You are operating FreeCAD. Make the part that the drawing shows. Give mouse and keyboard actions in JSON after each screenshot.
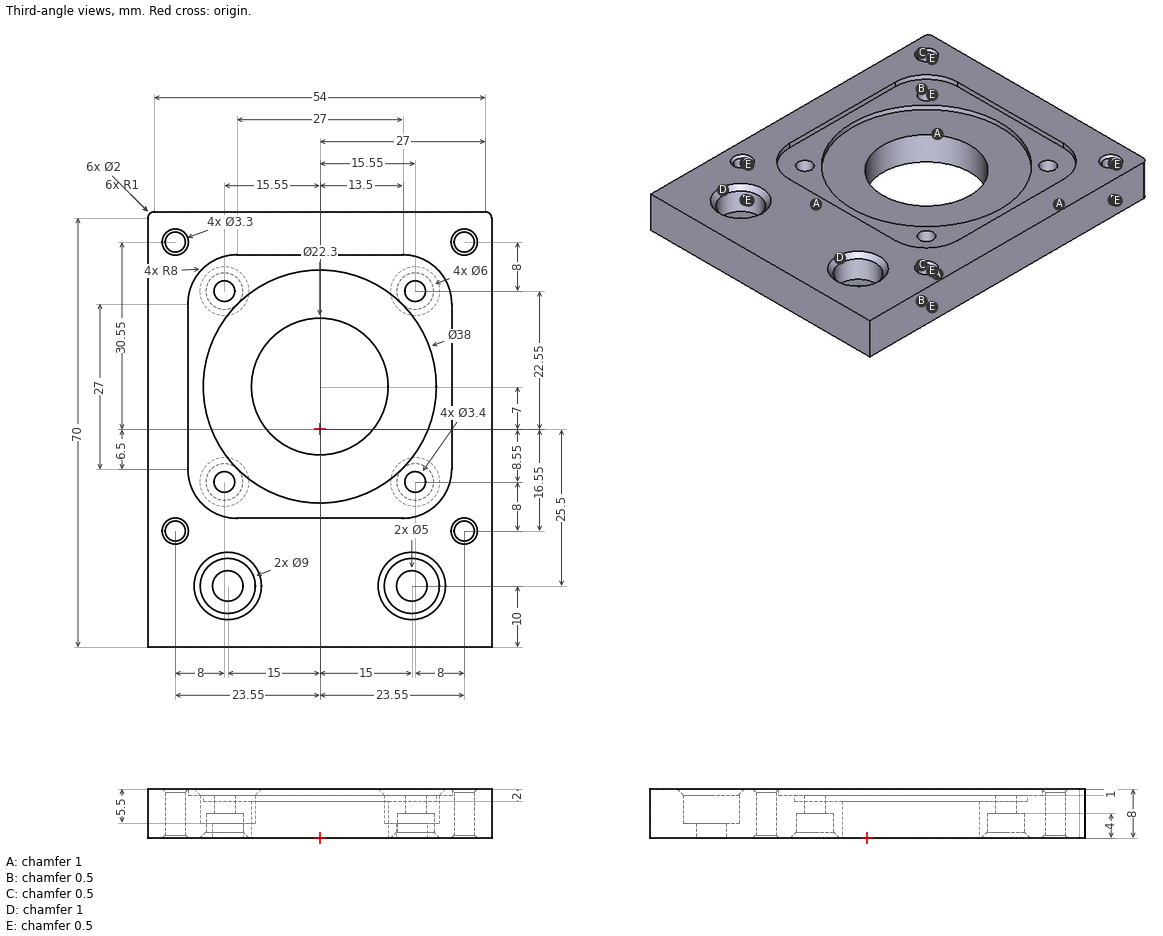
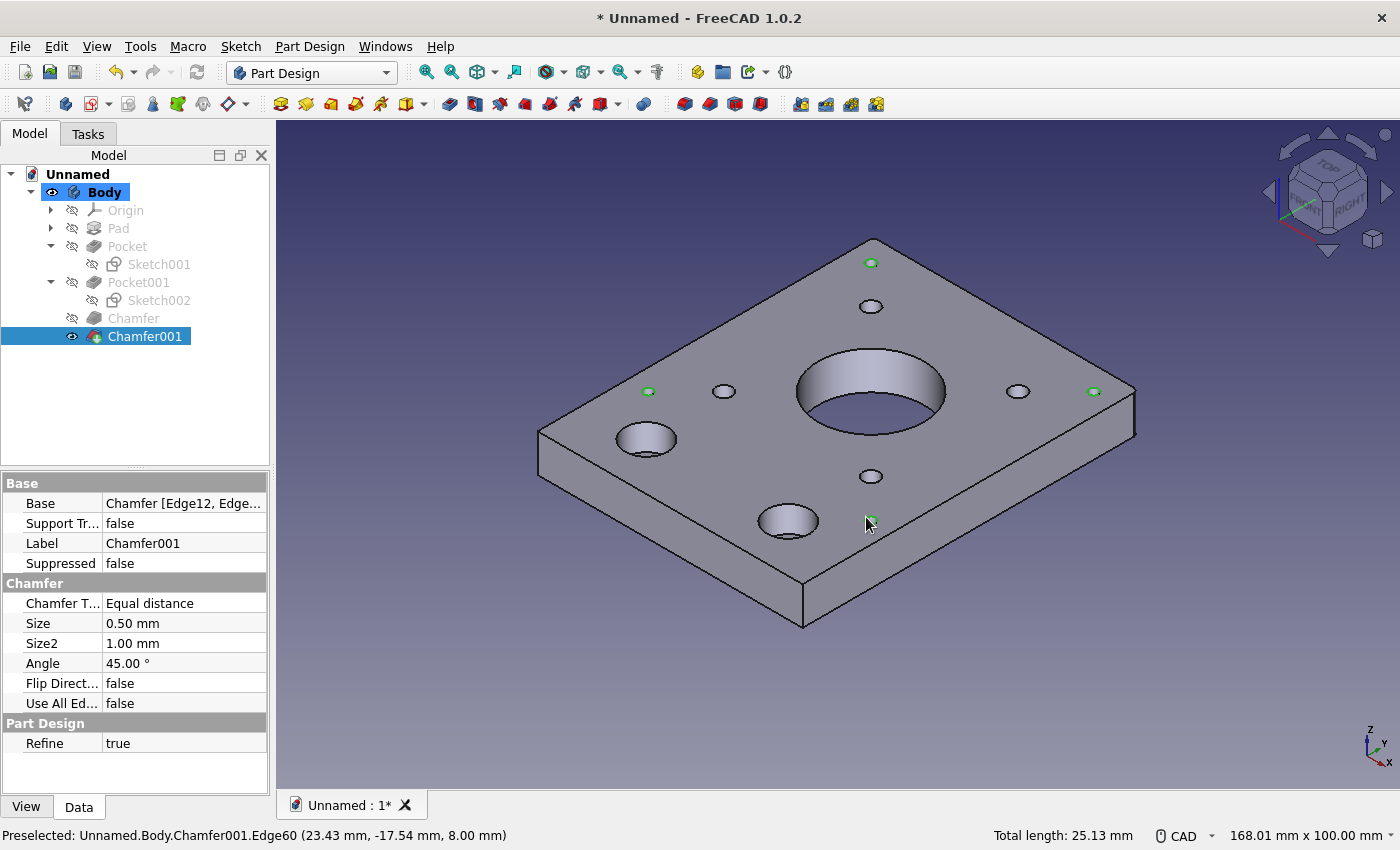
{"action": "left_click", "coordinate": [710, 104]}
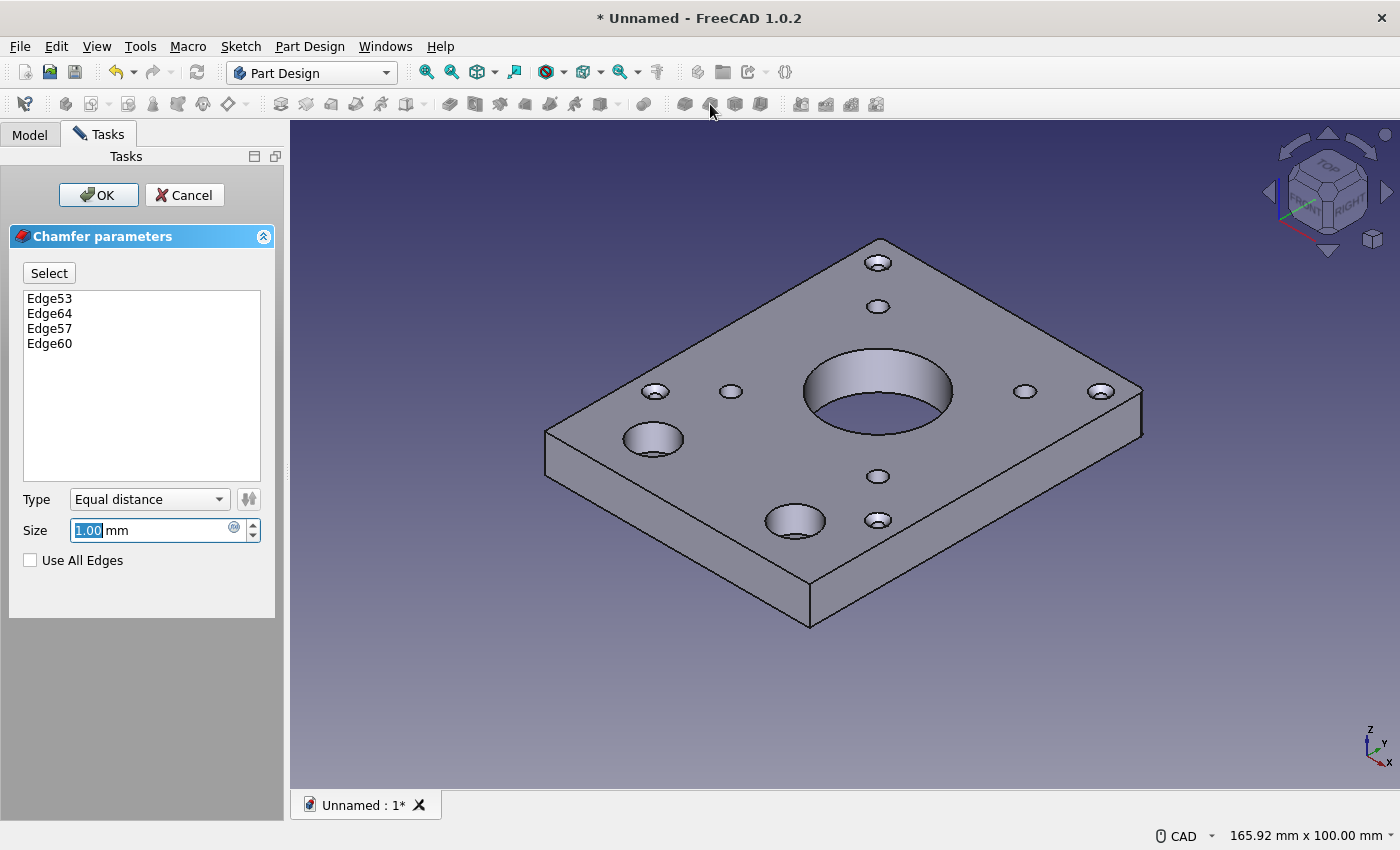
{"action": "type", "text": "0.5"}
{"action": "key", "text": "Tab"}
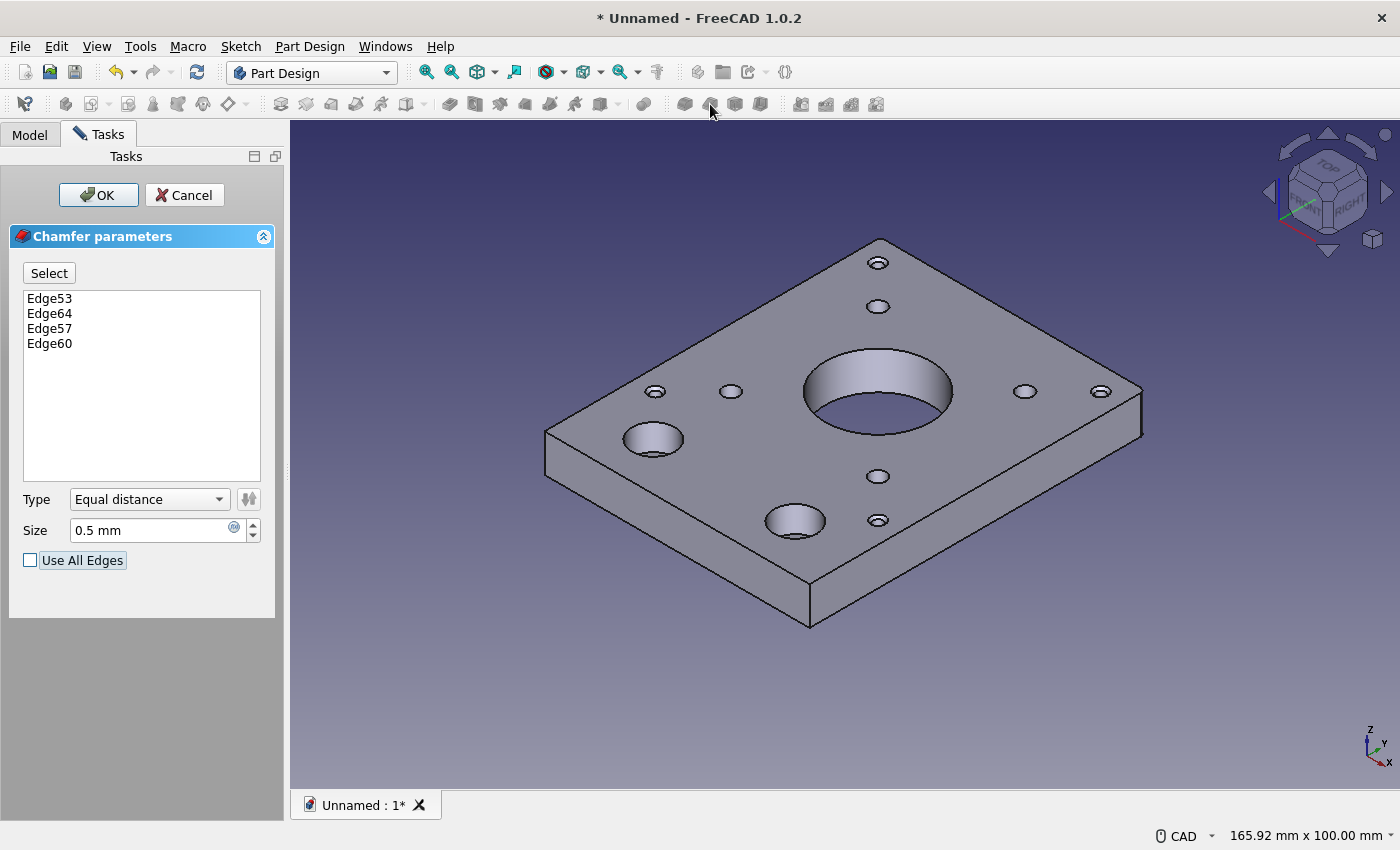
{"action": "left_click", "coordinate": [99, 195]}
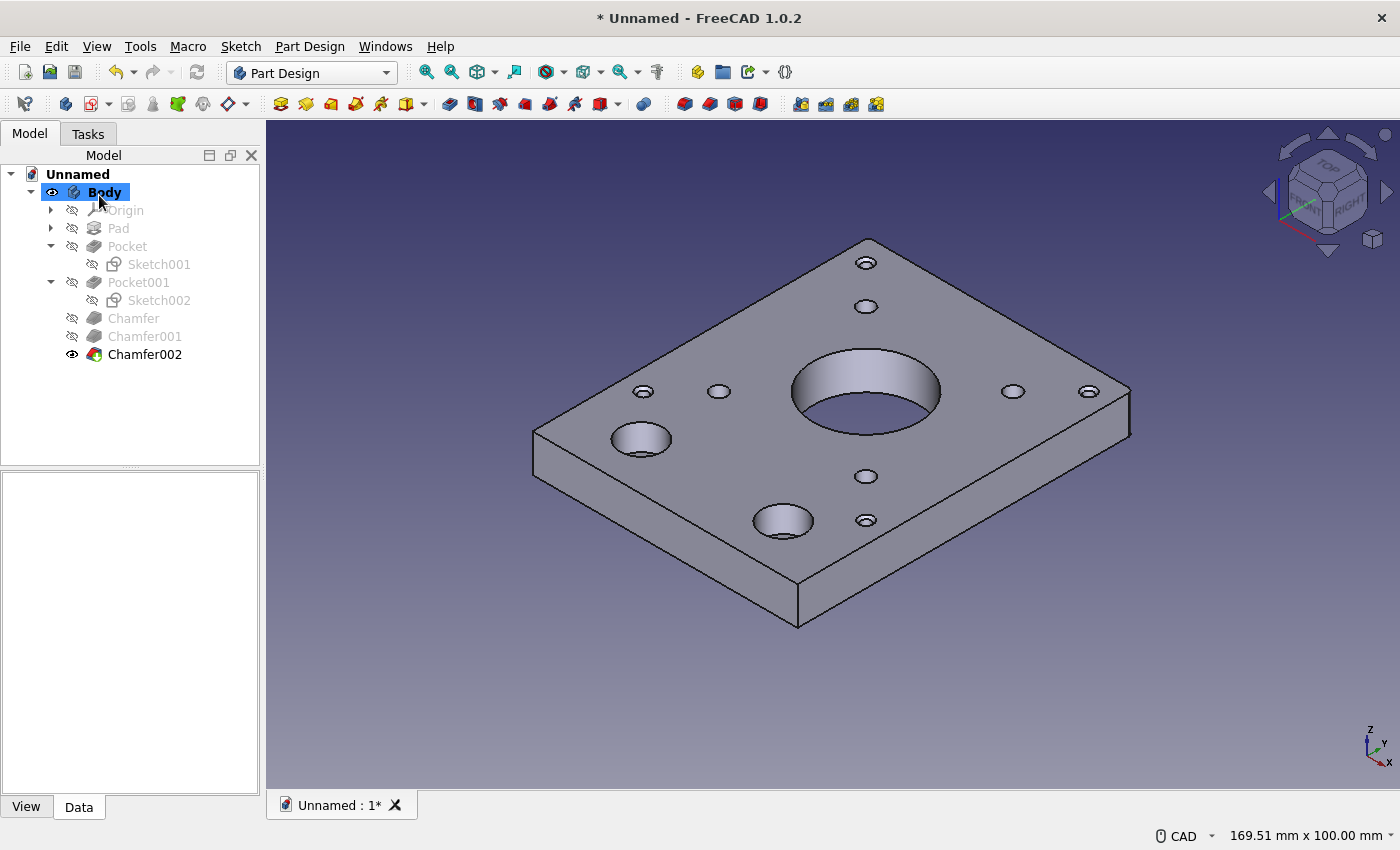
{"action": "left_click", "coordinate": [737, 465]}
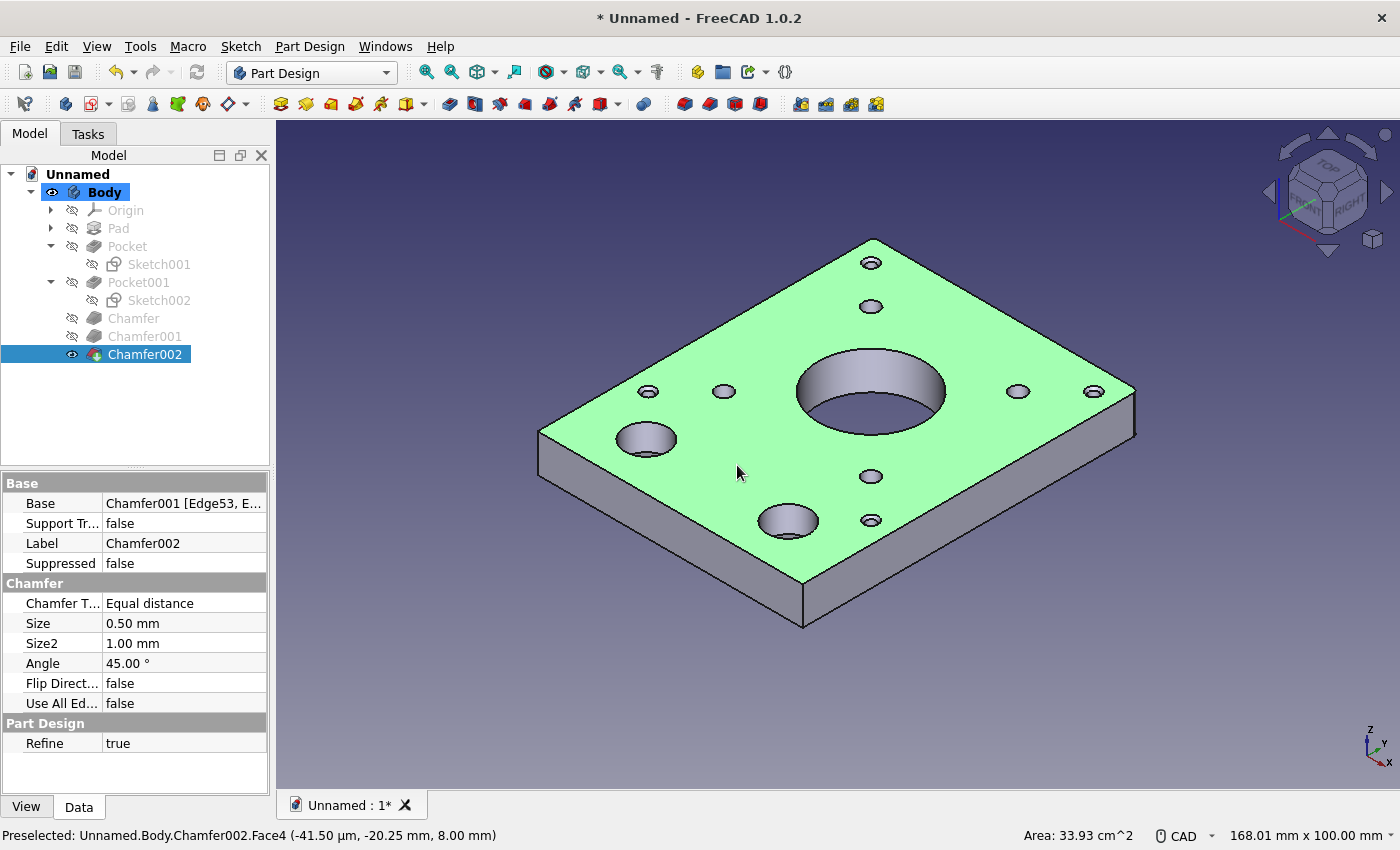
{"action": "left_click", "coordinate": [90, 104]}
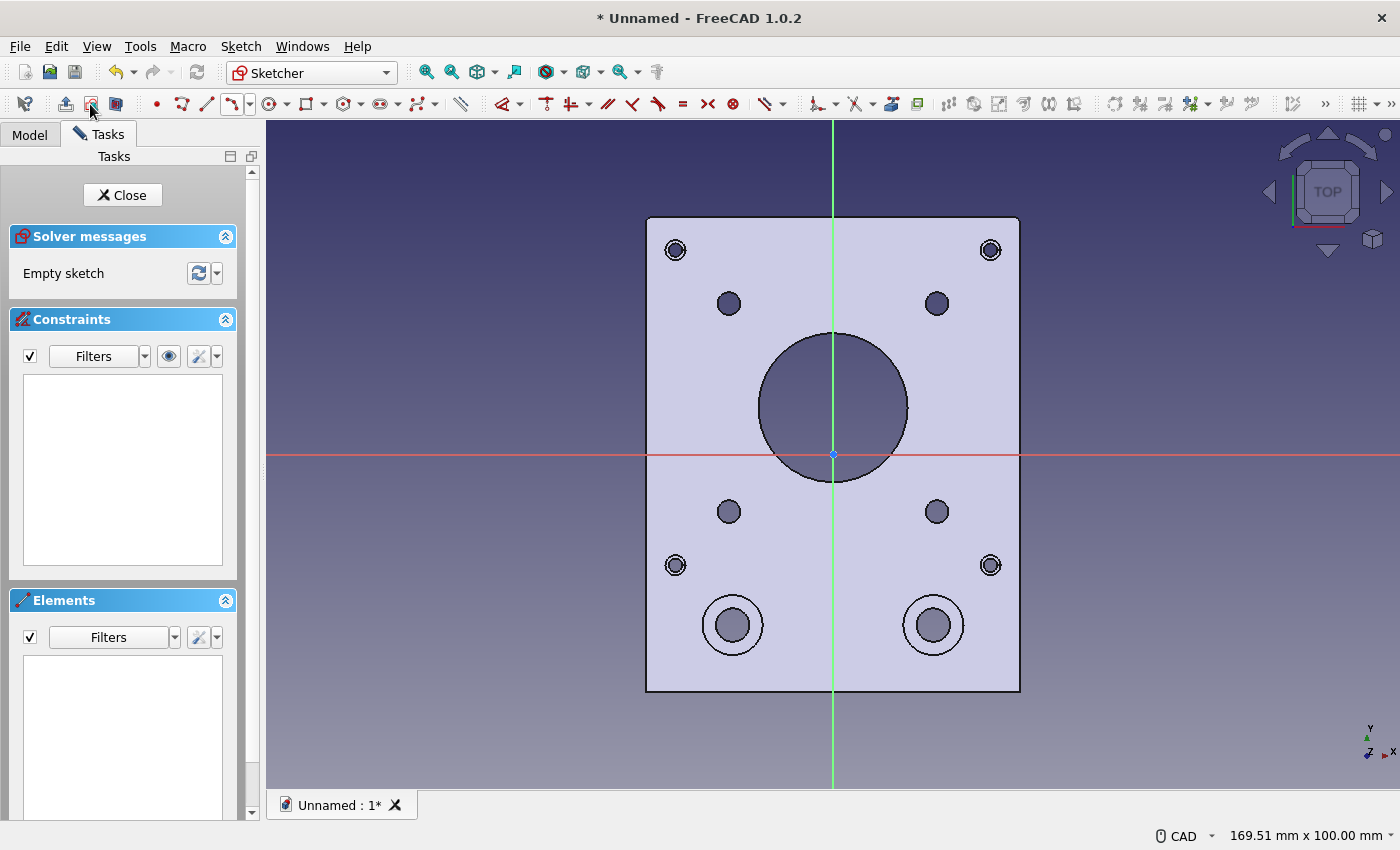
{"action": "scroll", "coordinate": [916, 351], "scroll_direction": "up", "scroll_amount": 3}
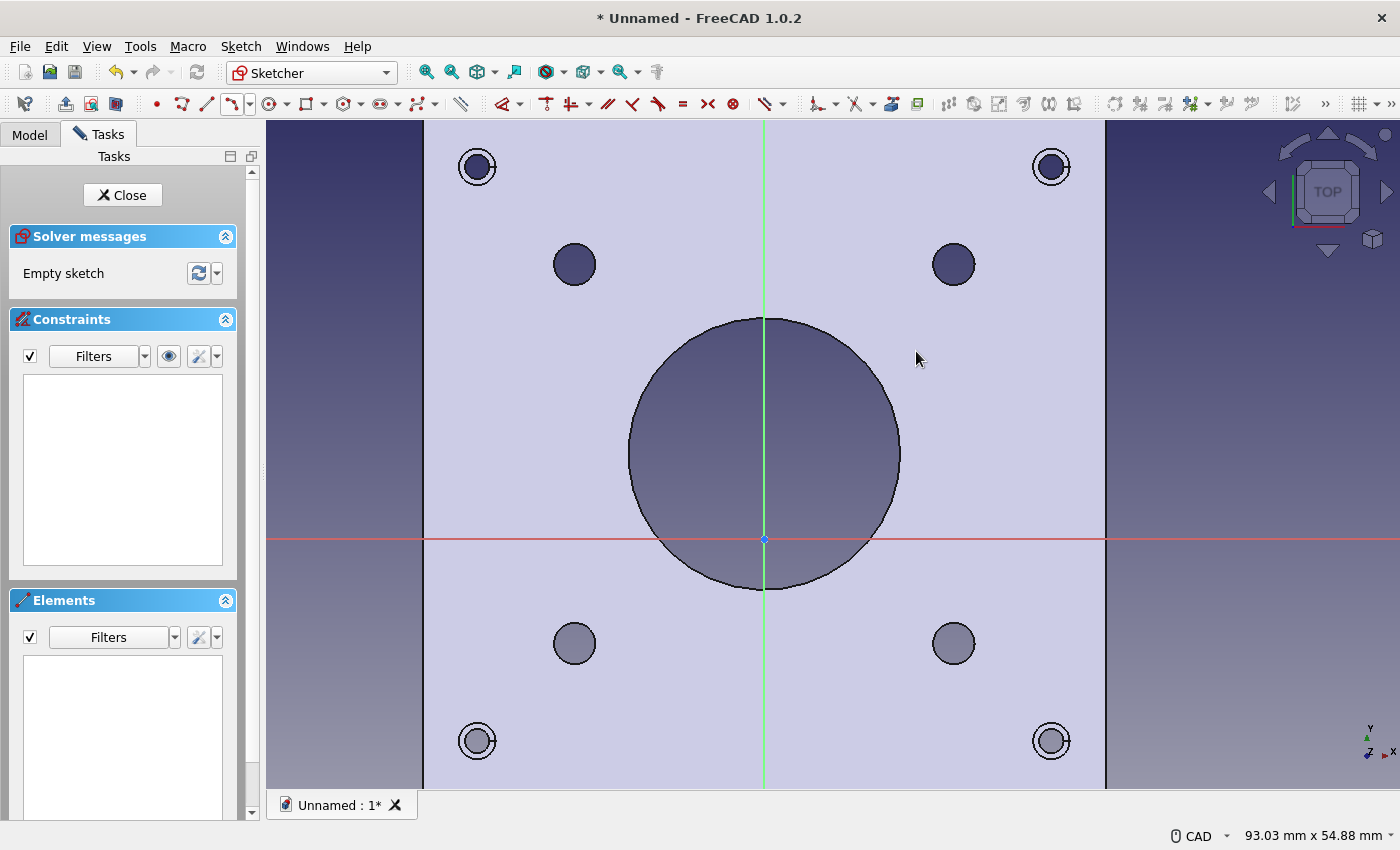
{"action": "left_click", "coordinate": [268, 104]}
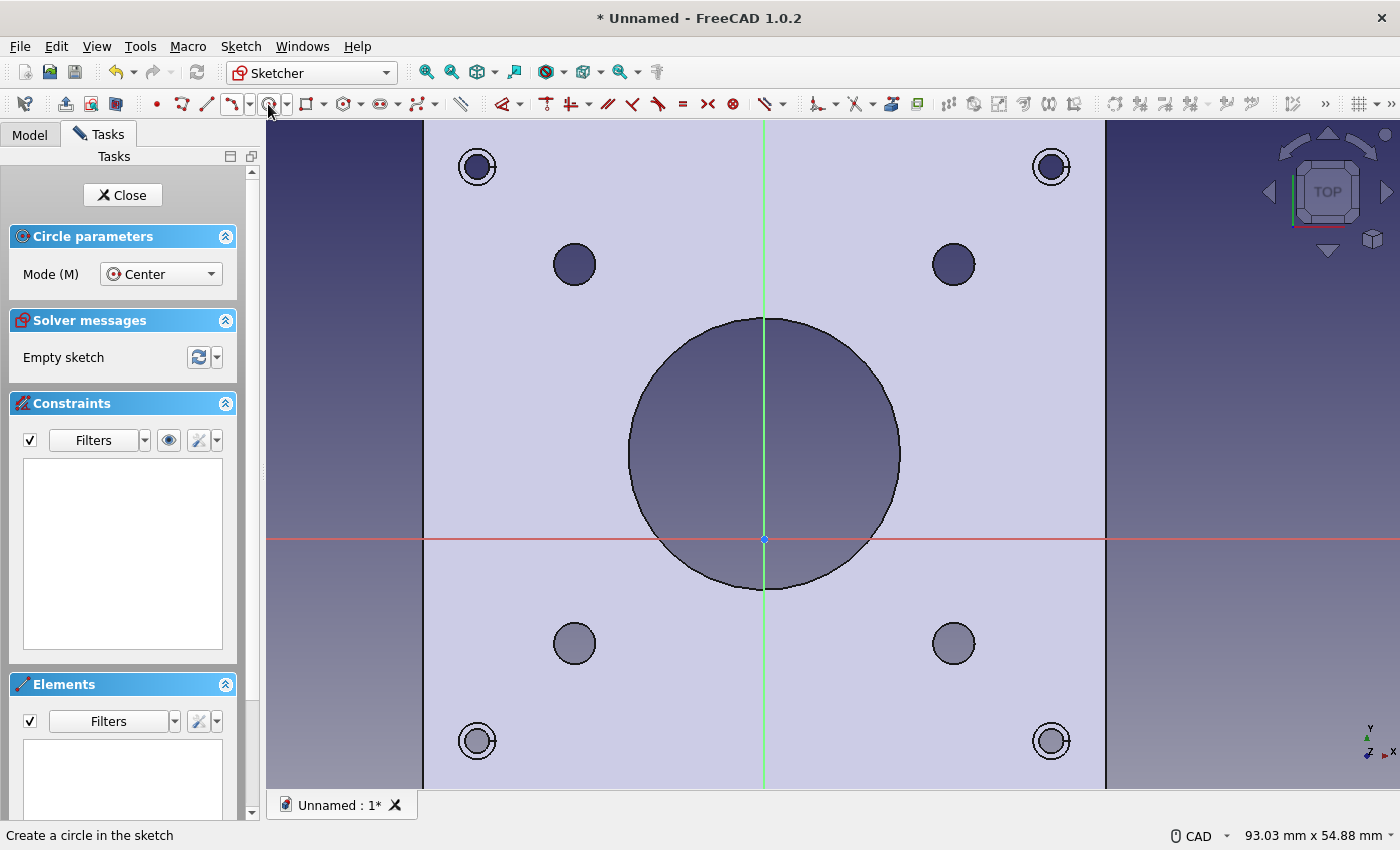
{"action": "left_click", "coordinate": [764, 454]}
{"action": "left_click", "coordinate": [928, 290]}
{"action": "key", "text": "Escape"}